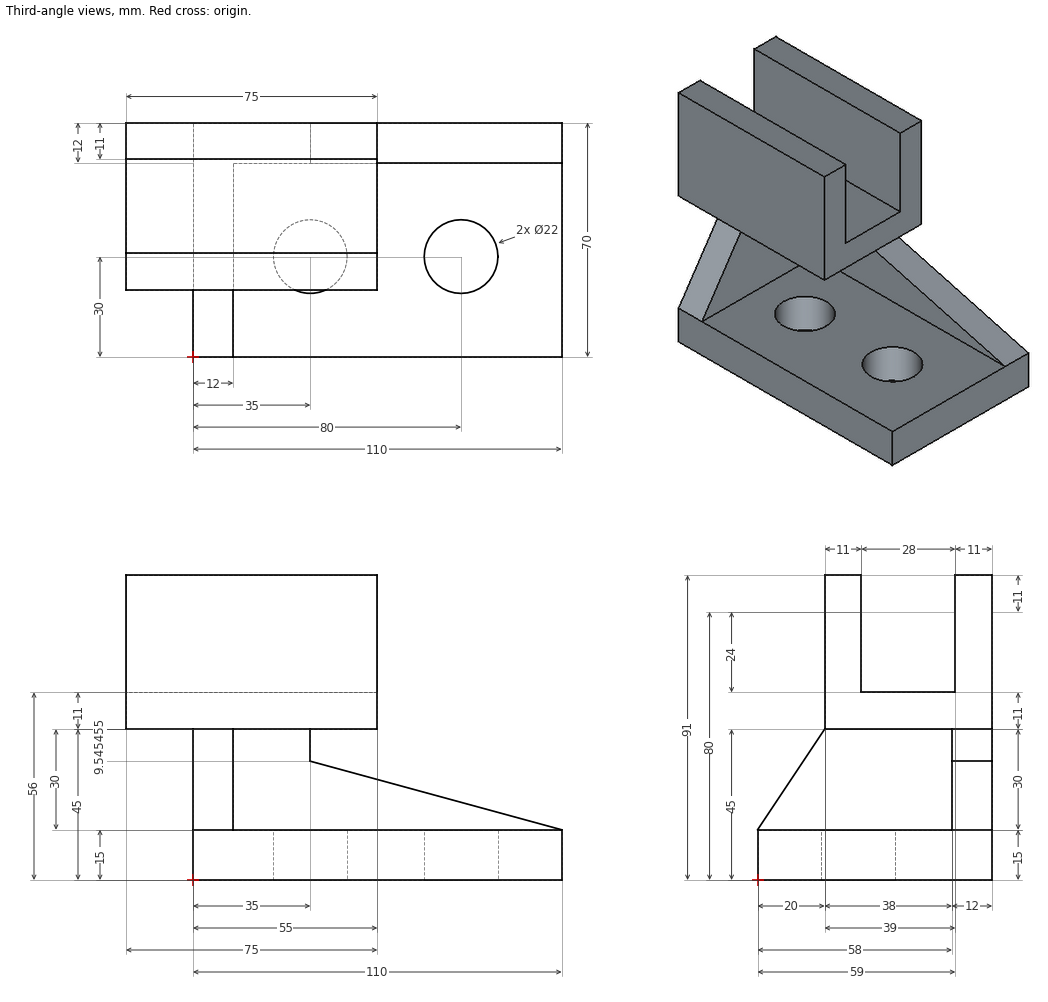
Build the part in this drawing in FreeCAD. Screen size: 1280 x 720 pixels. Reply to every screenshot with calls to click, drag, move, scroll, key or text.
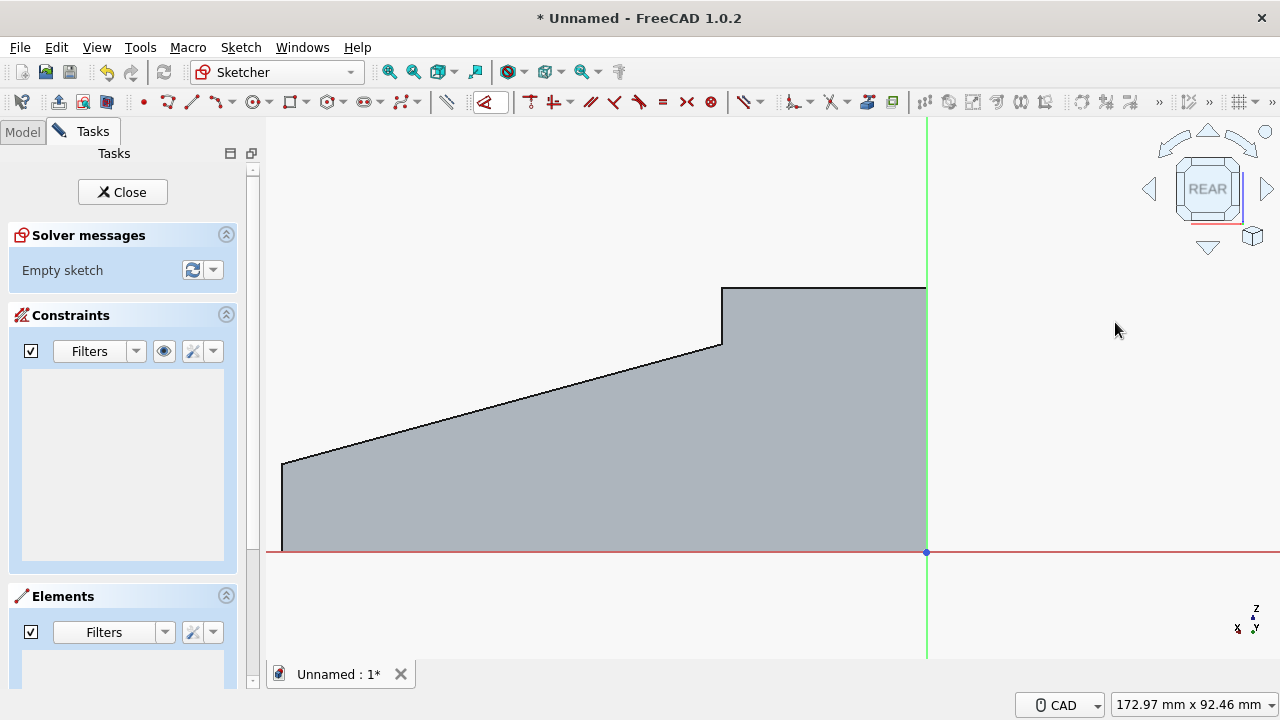
key(g)
key(r)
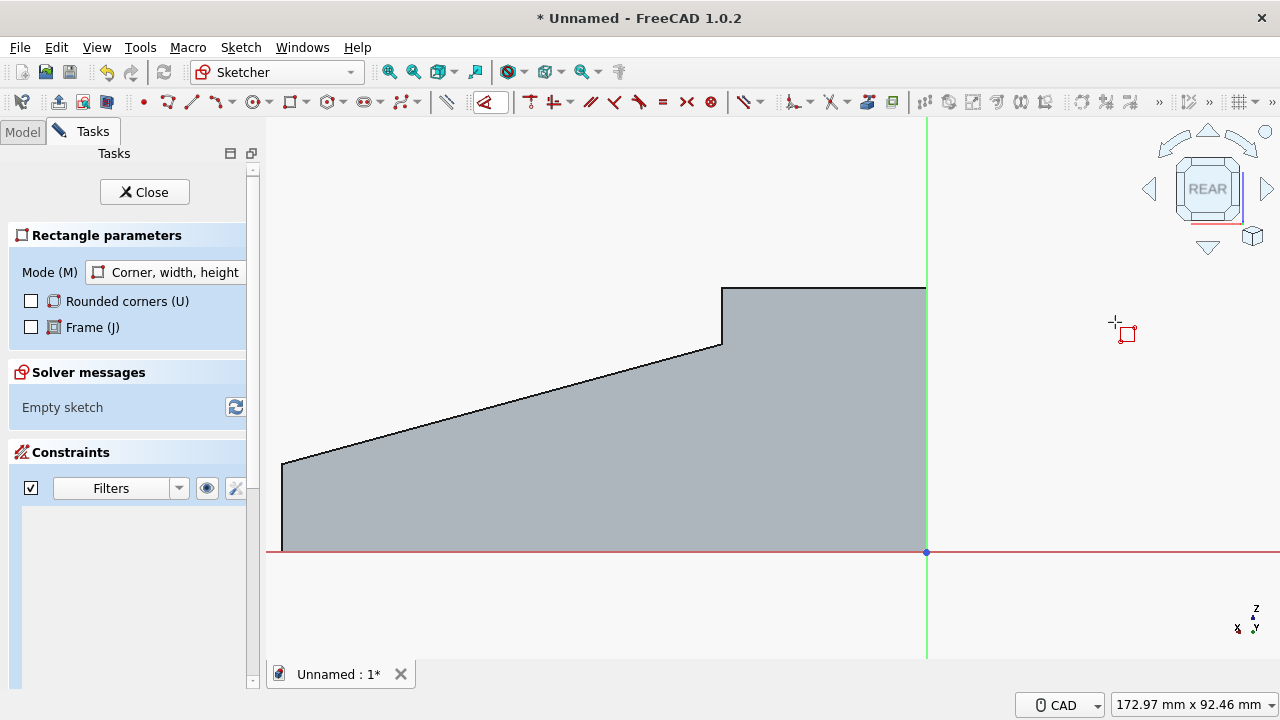
click(604, 224)
move(1044, 288)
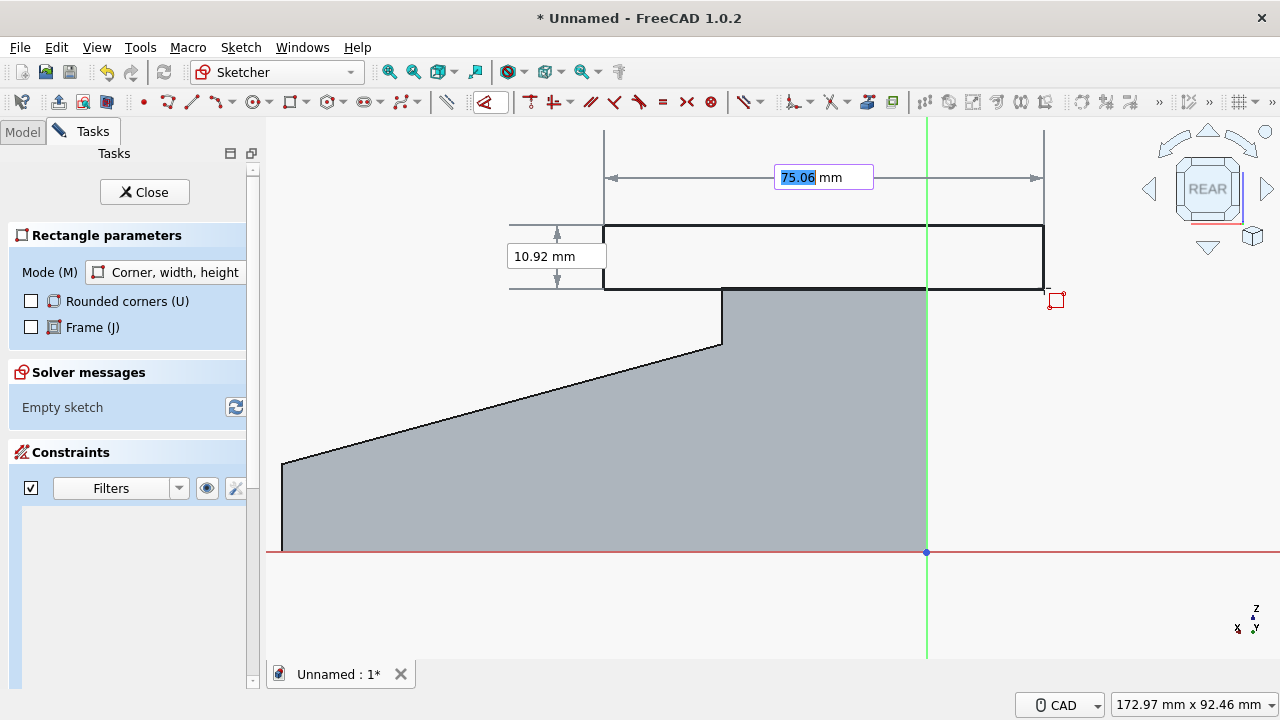
text(75)
key(Tab)
text(11)
key(Return)
key(Escape)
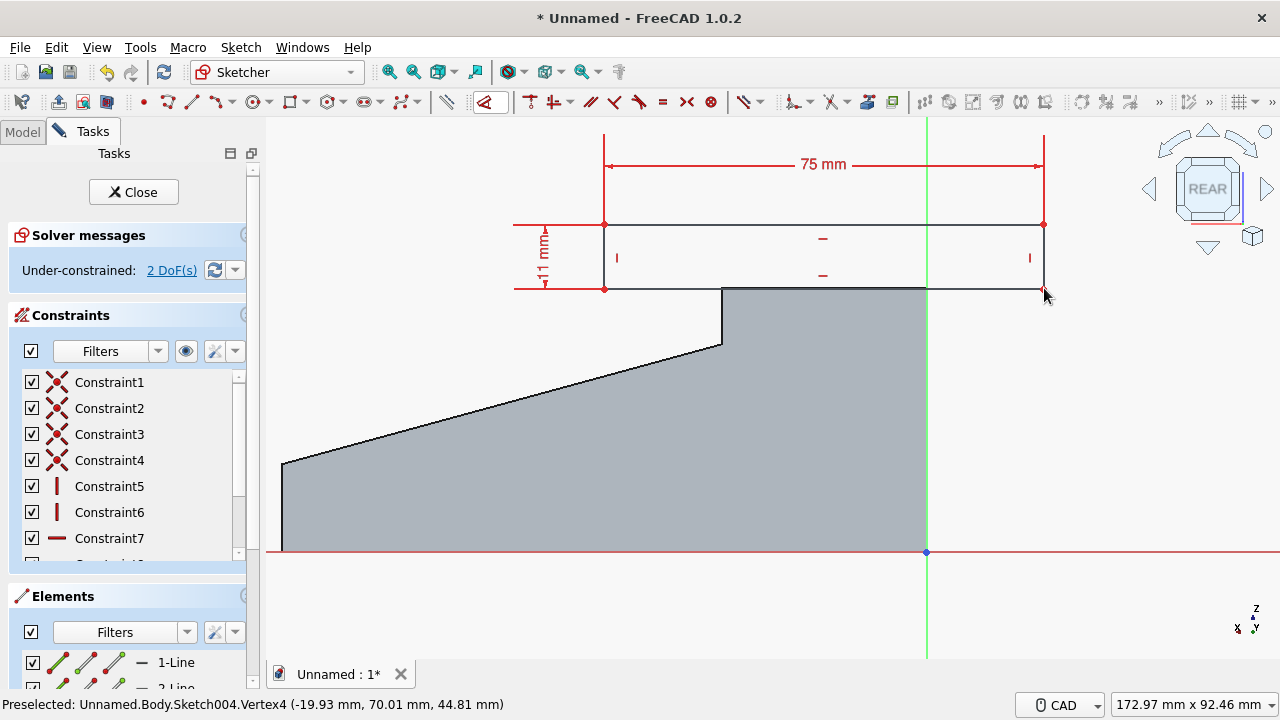
click(604, 225)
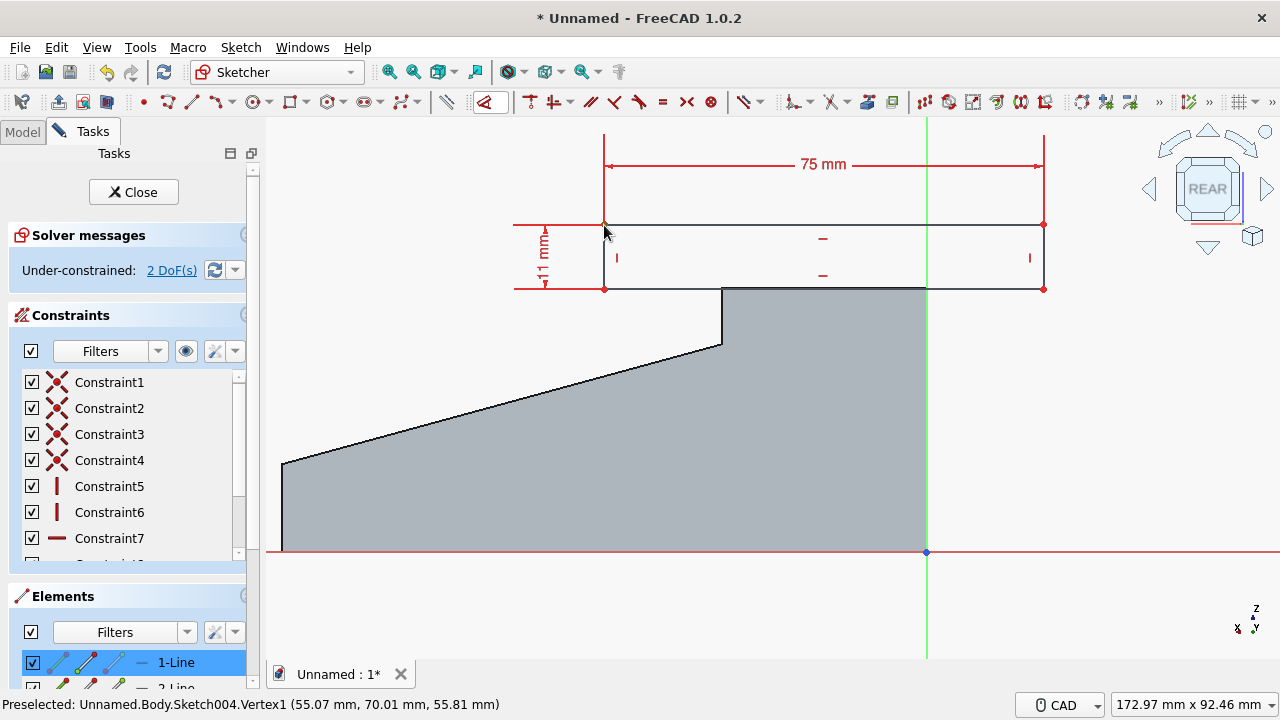
click(502, 102)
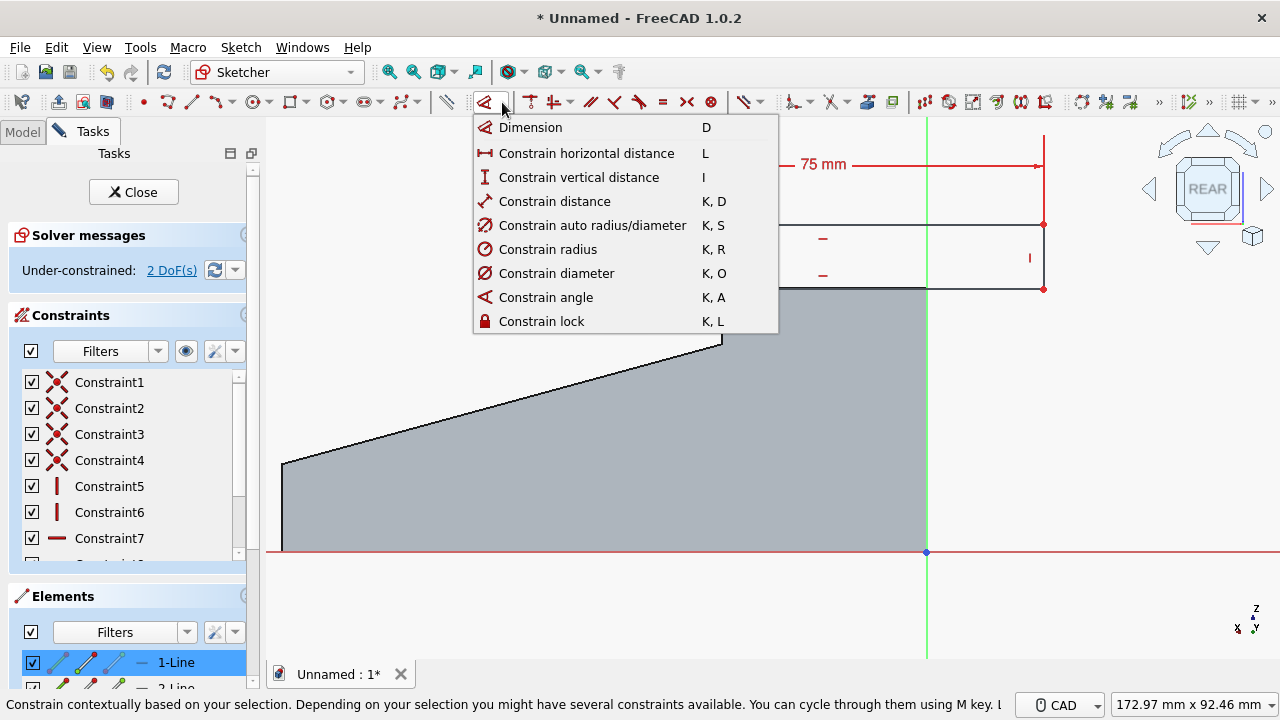
click(626, 153)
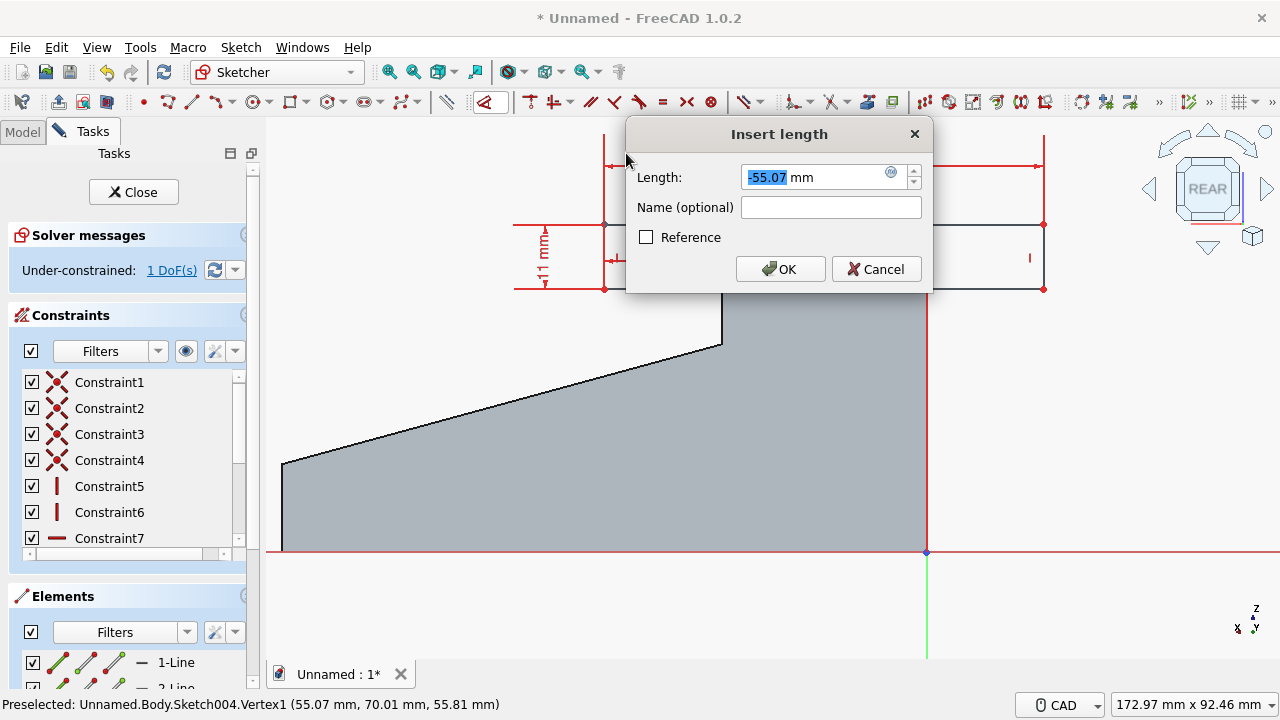
text(-55)
key(Return)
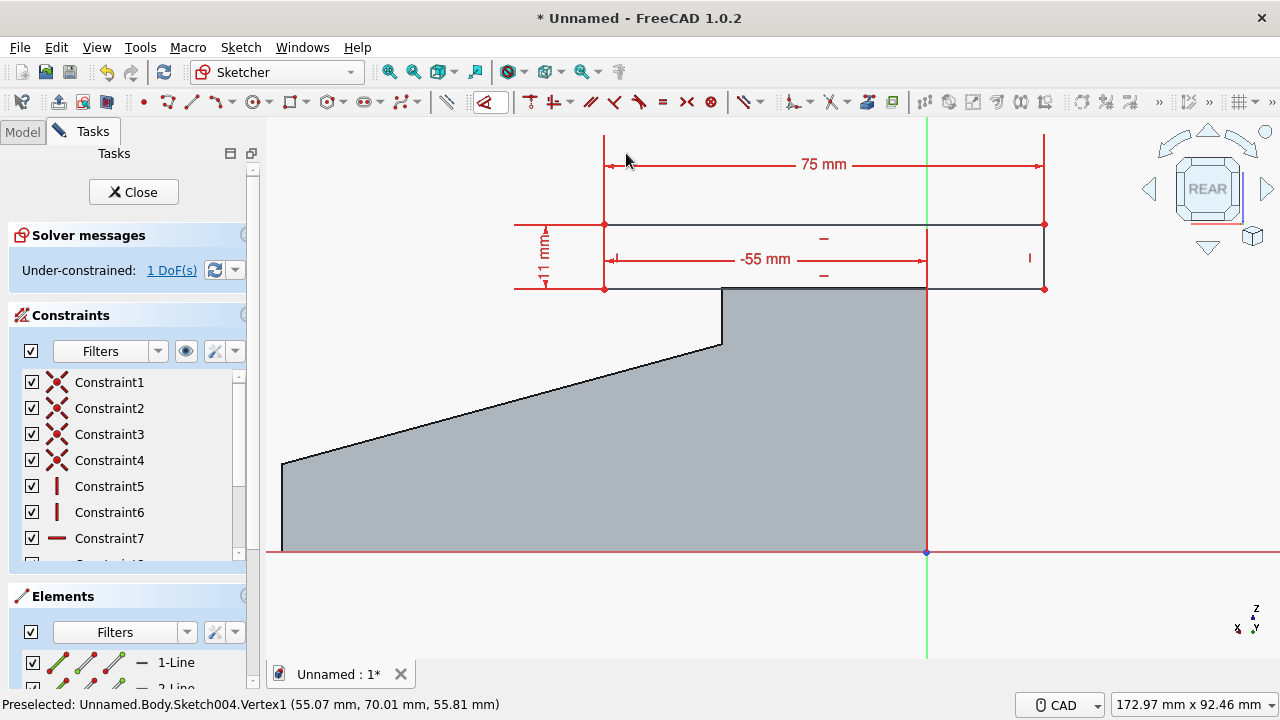
click(604, 225)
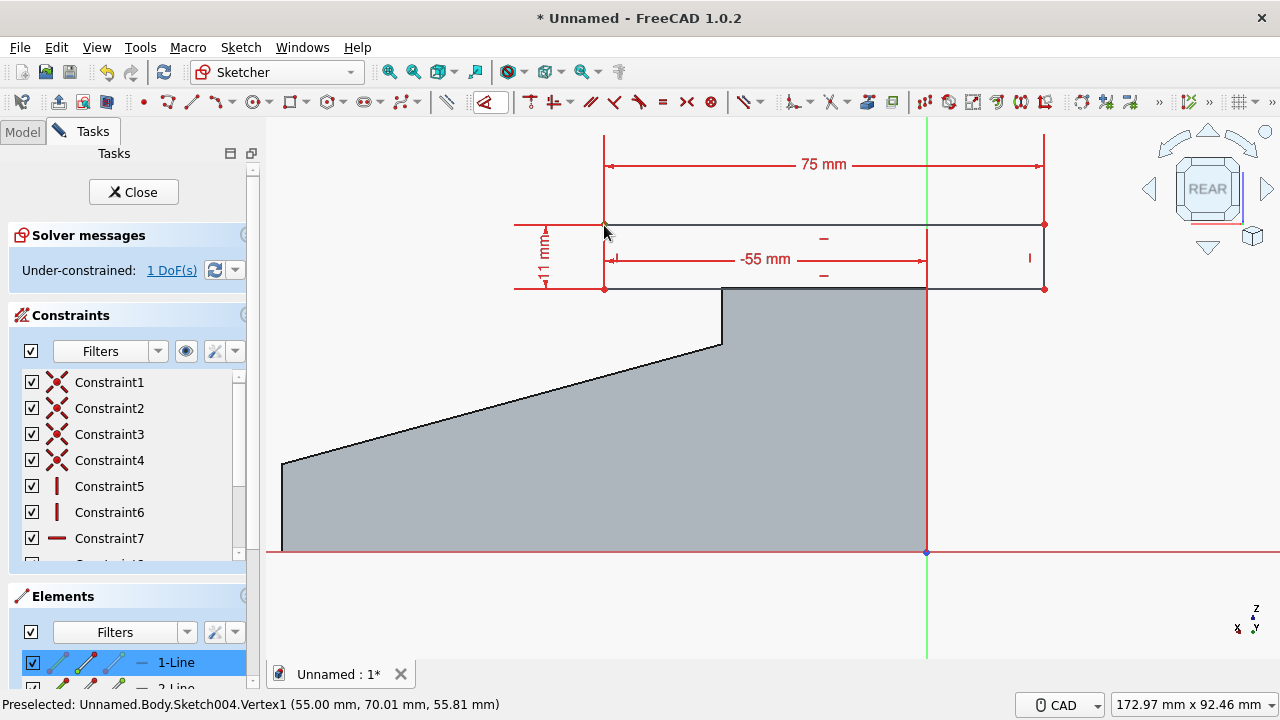
click(502, 102)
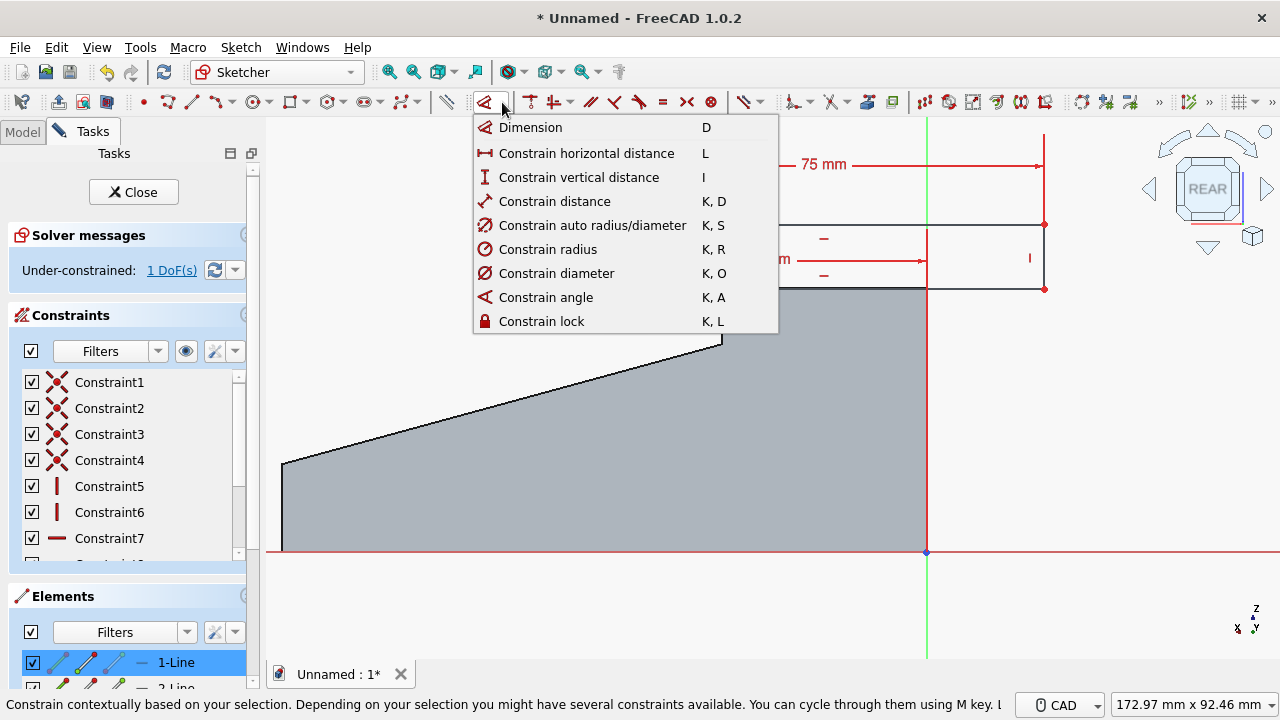
click(626, 177)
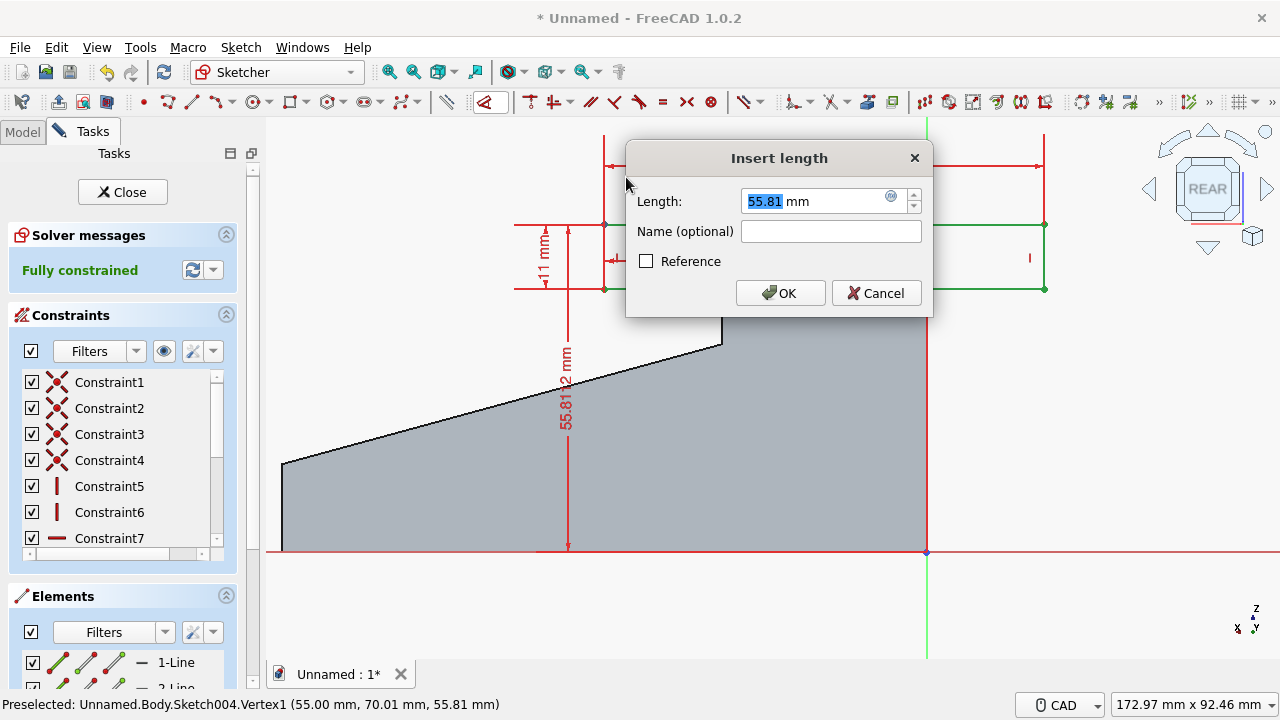
text(56)
key(Return)